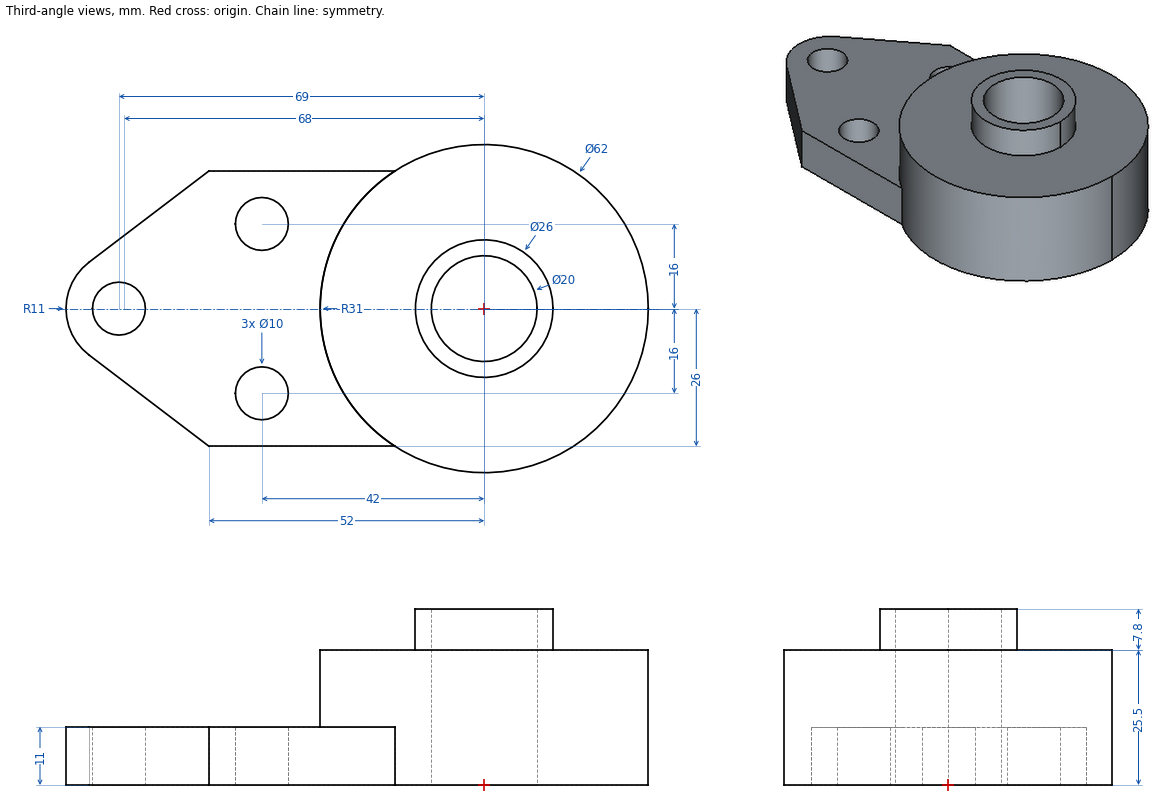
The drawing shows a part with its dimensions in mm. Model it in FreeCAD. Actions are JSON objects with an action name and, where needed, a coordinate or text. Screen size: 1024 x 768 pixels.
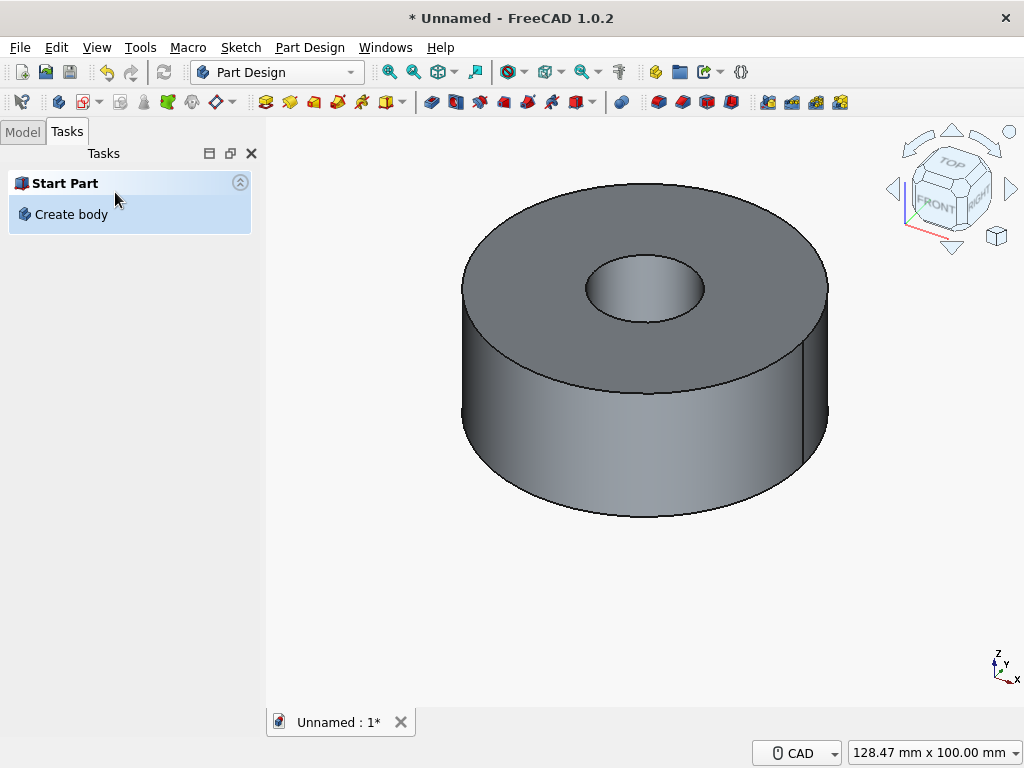
{"action": "left_click", "coordinate": [84, 102]}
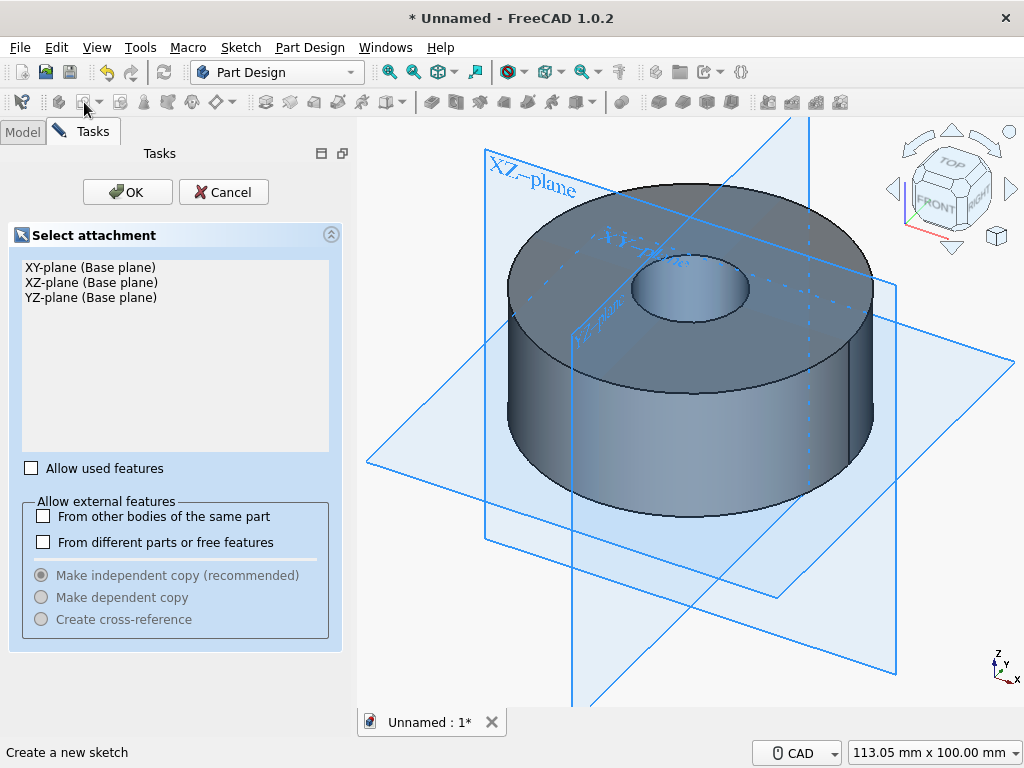
{"action": "left_click", "coordinate": [82, 268]}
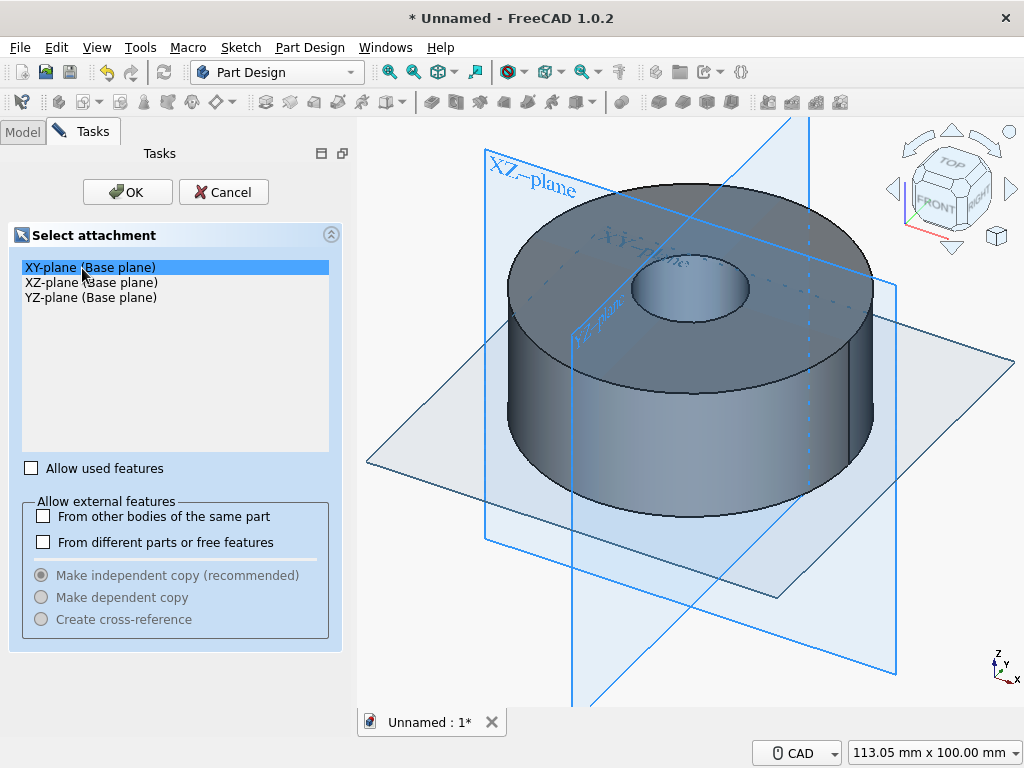
{"action": "left_click", "coordinate": [128, 192]}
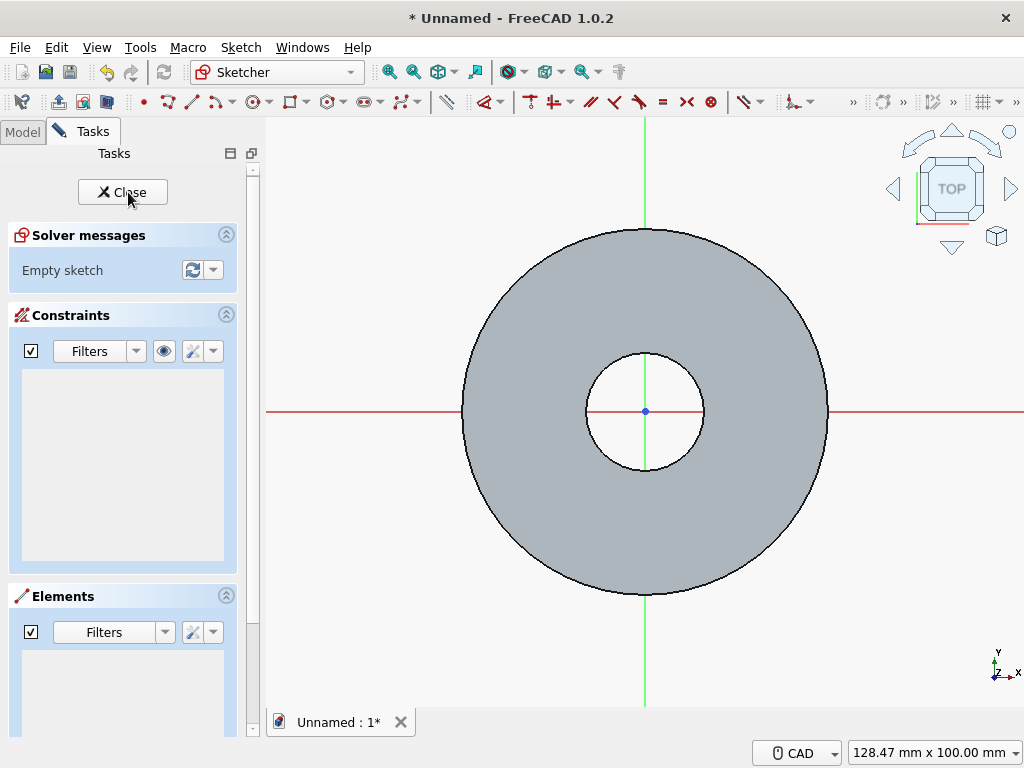
{"action": "left_click", "coordinate": [108, 102]}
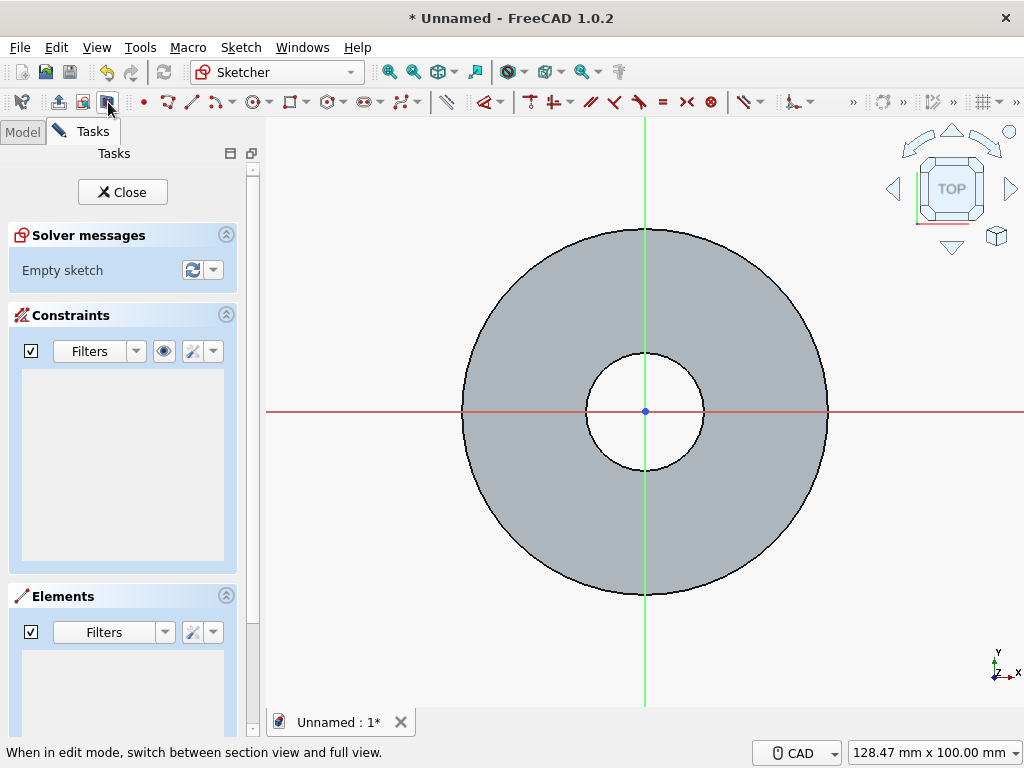
{"action": "scroll", "coordinate": [859, 412], "scroll_direction": "down", "scroll_amount": 2}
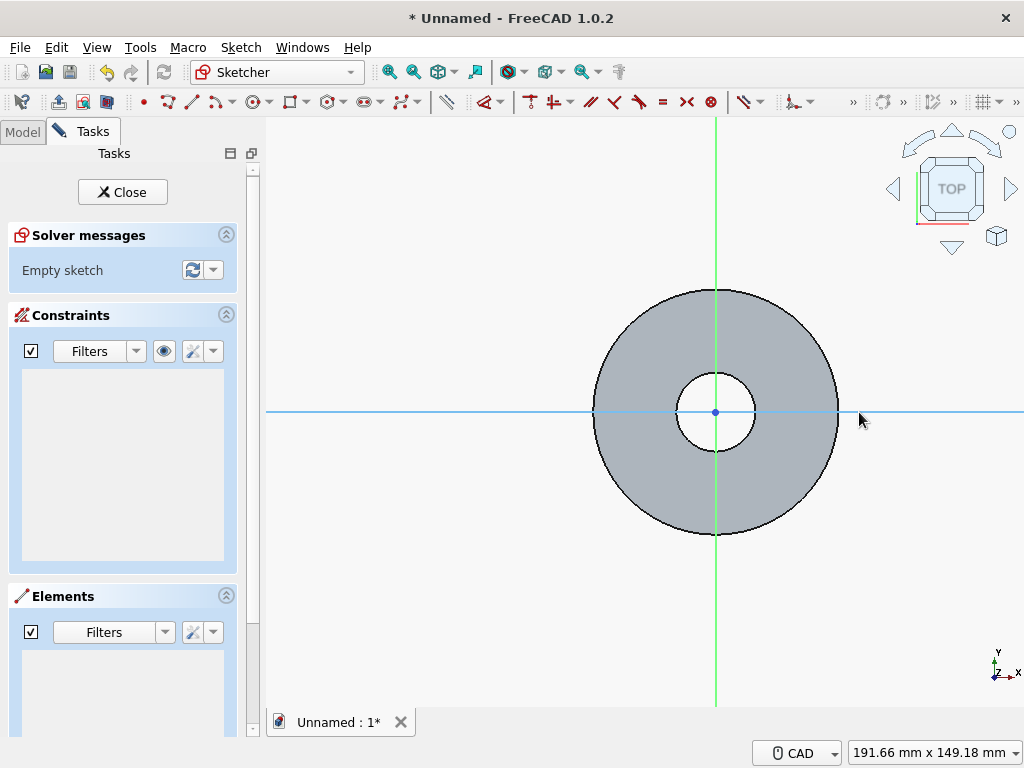
{"action": "left_click", "coordinate": [168, 102]}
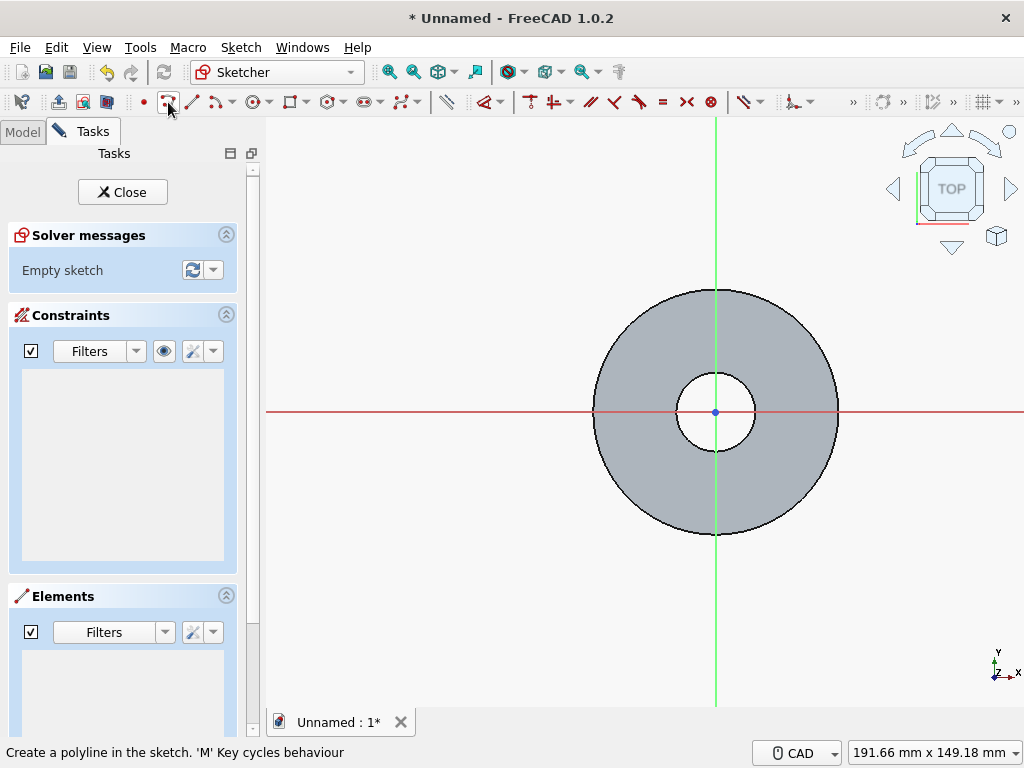
{"action": "left_click", "coordinate": [649, 515]}
{"action": "left_click", "coordinate": [510, 515]}
{"action": "left_click", "coordinate": [421, 447]}
{"action": "right_click", "coordinate": [421, 447]}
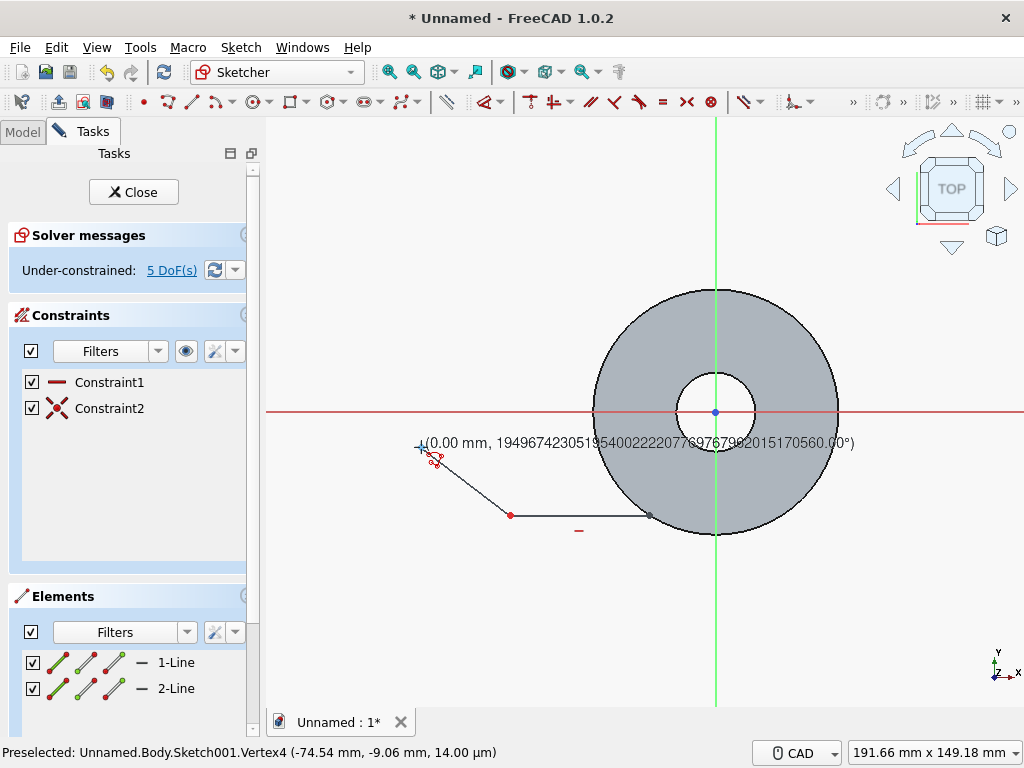
{"action": "left_click", "coordinate": [421, 378]}
{"action": "left_click", "coordinate": [510, 309]}
{"action": "left_click", "coordinate": [649, 309]}
{"action": "right_click", "coordinate": [649, 309]}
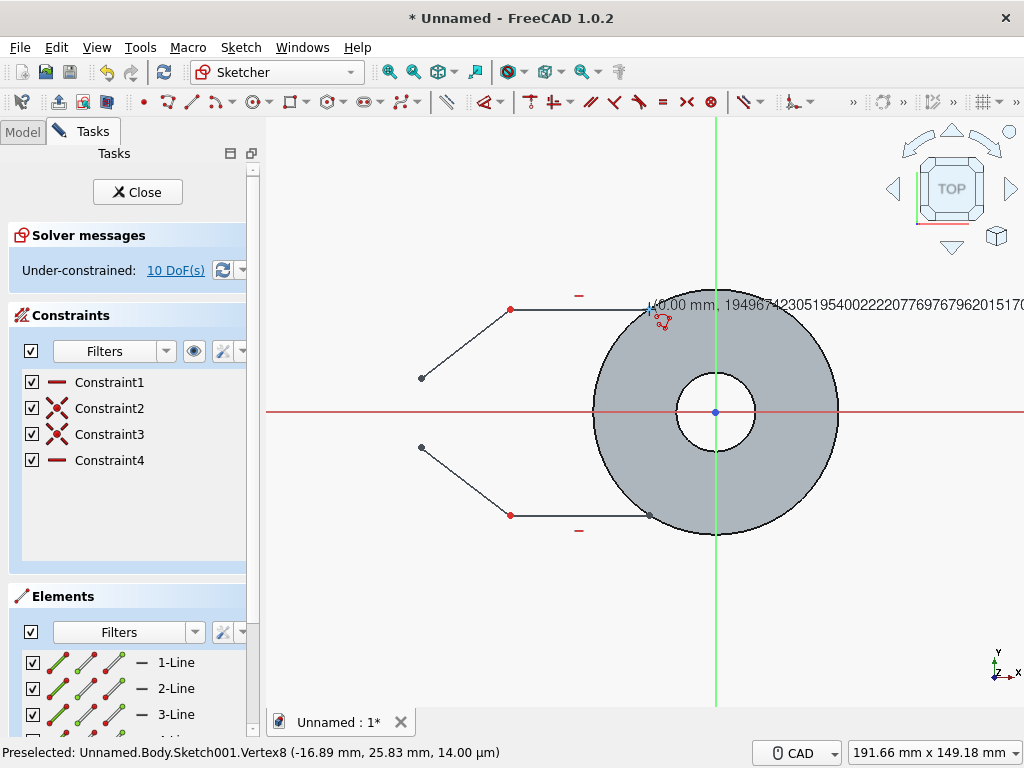
{"action": "left_click", "coordinate": [234, 102]}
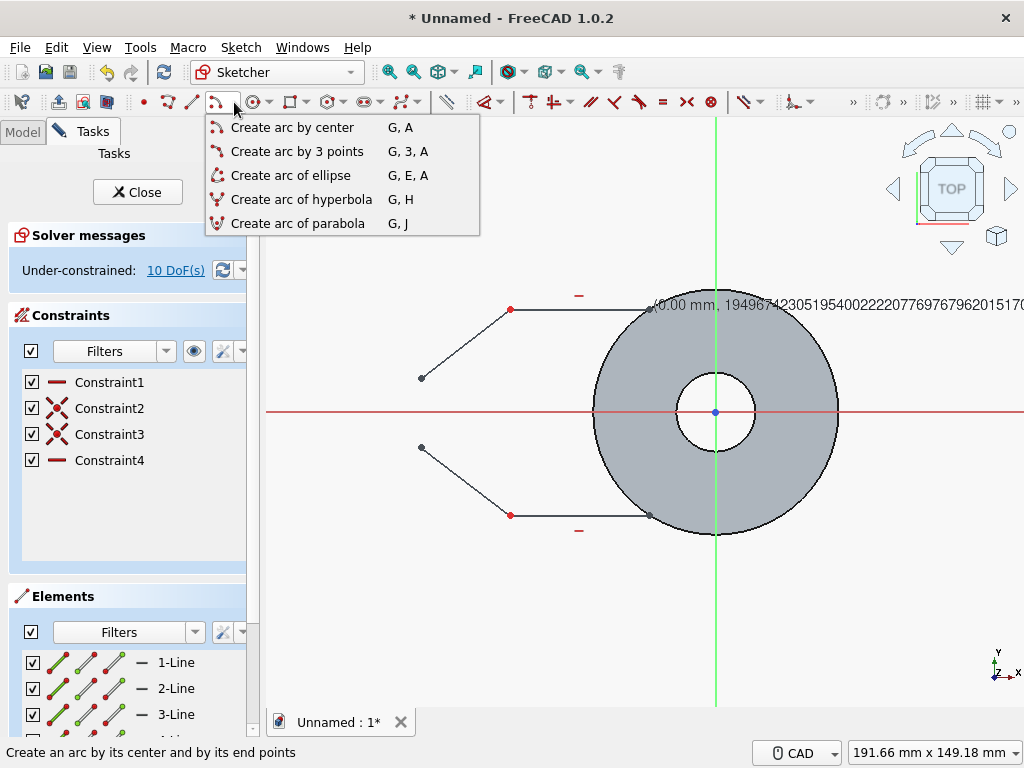
{"action": "left_click", "coordinate": [342, 151]}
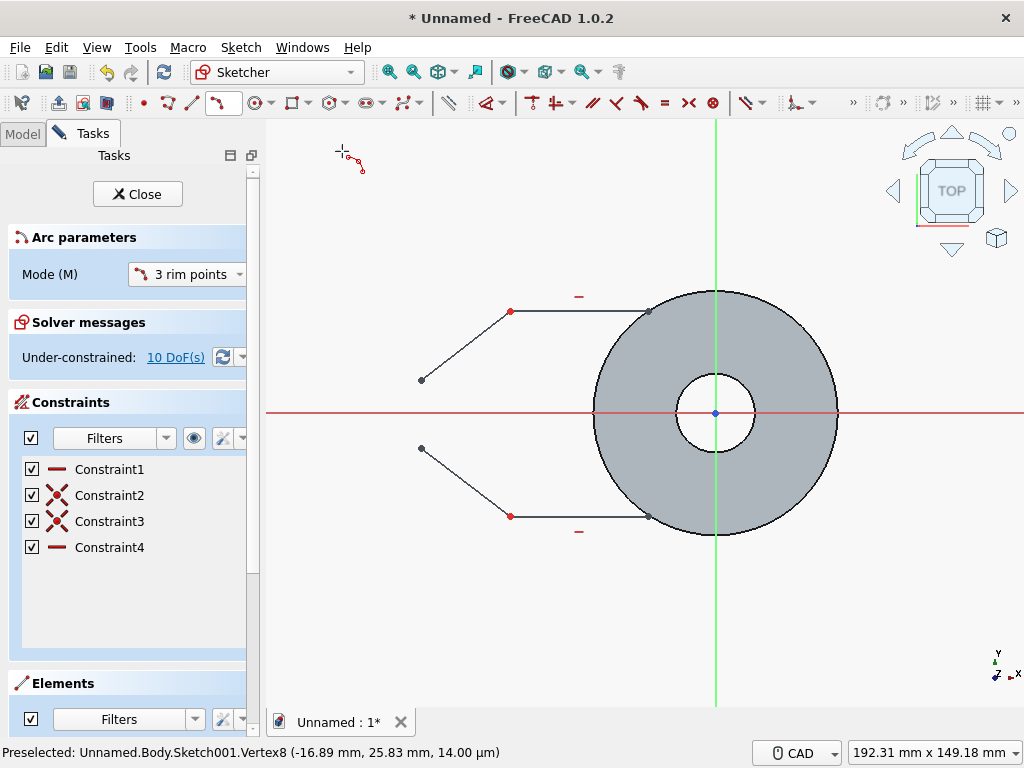
{"action": "left_click", "coordinate": [422, 449]}
{"action": "left_click", "coordinate": [422, 380]}
{"action": "left_click", "coordinate": [407, 398]}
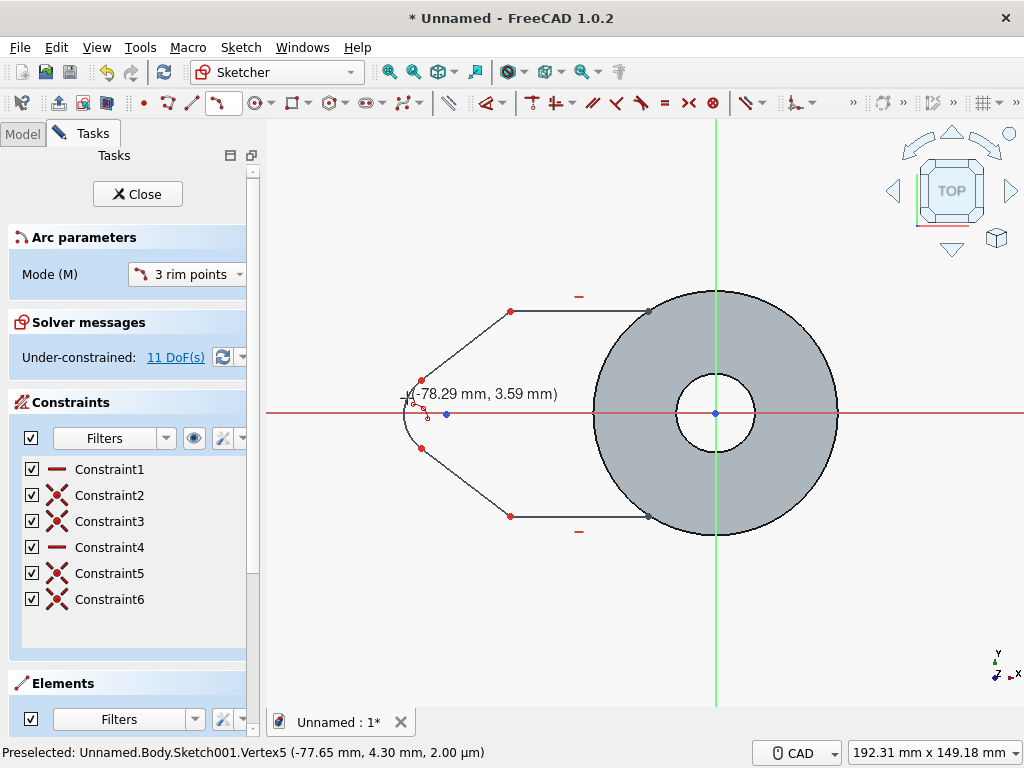
{"action": "left_click", "coordinate": [649, 311]}
{"action": "left_click", "coordinate": [649, 517]}
{"action": "left_click", "coordinate": [596, 389]}